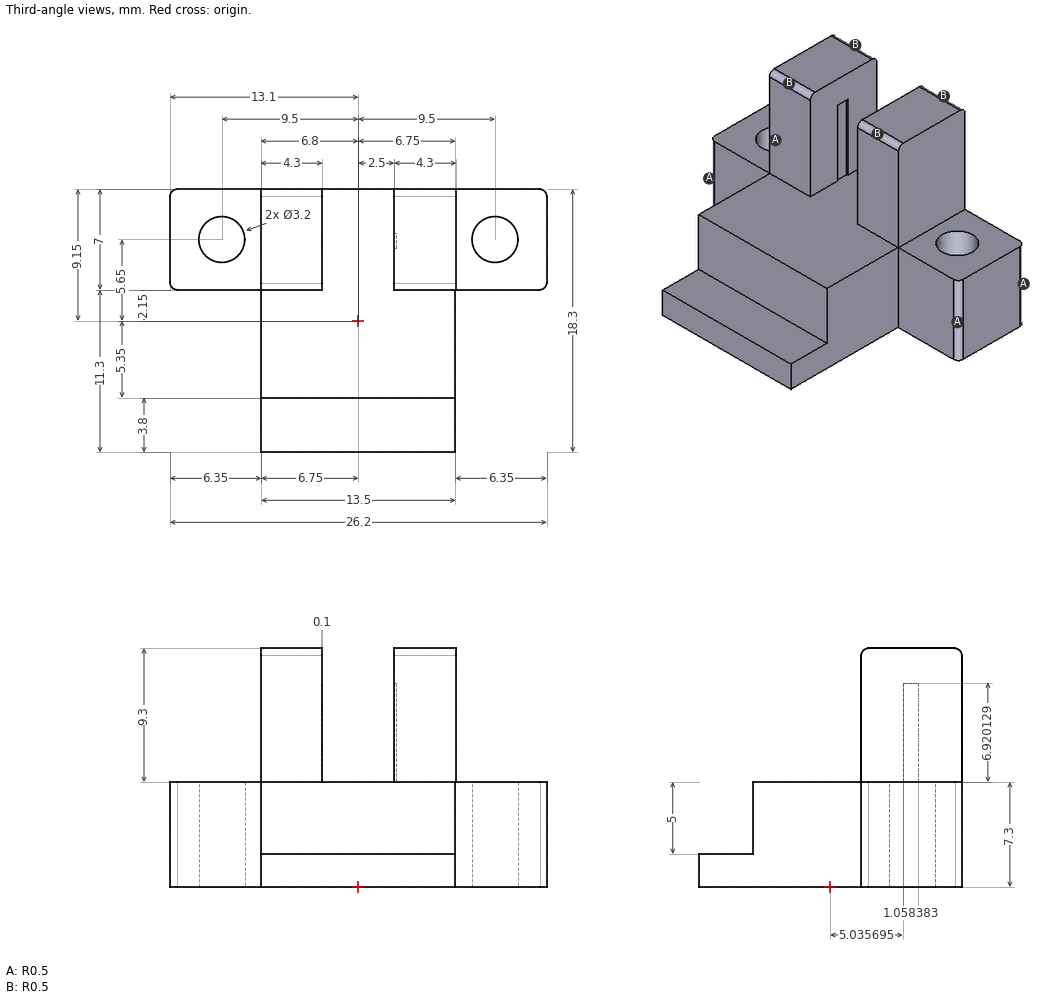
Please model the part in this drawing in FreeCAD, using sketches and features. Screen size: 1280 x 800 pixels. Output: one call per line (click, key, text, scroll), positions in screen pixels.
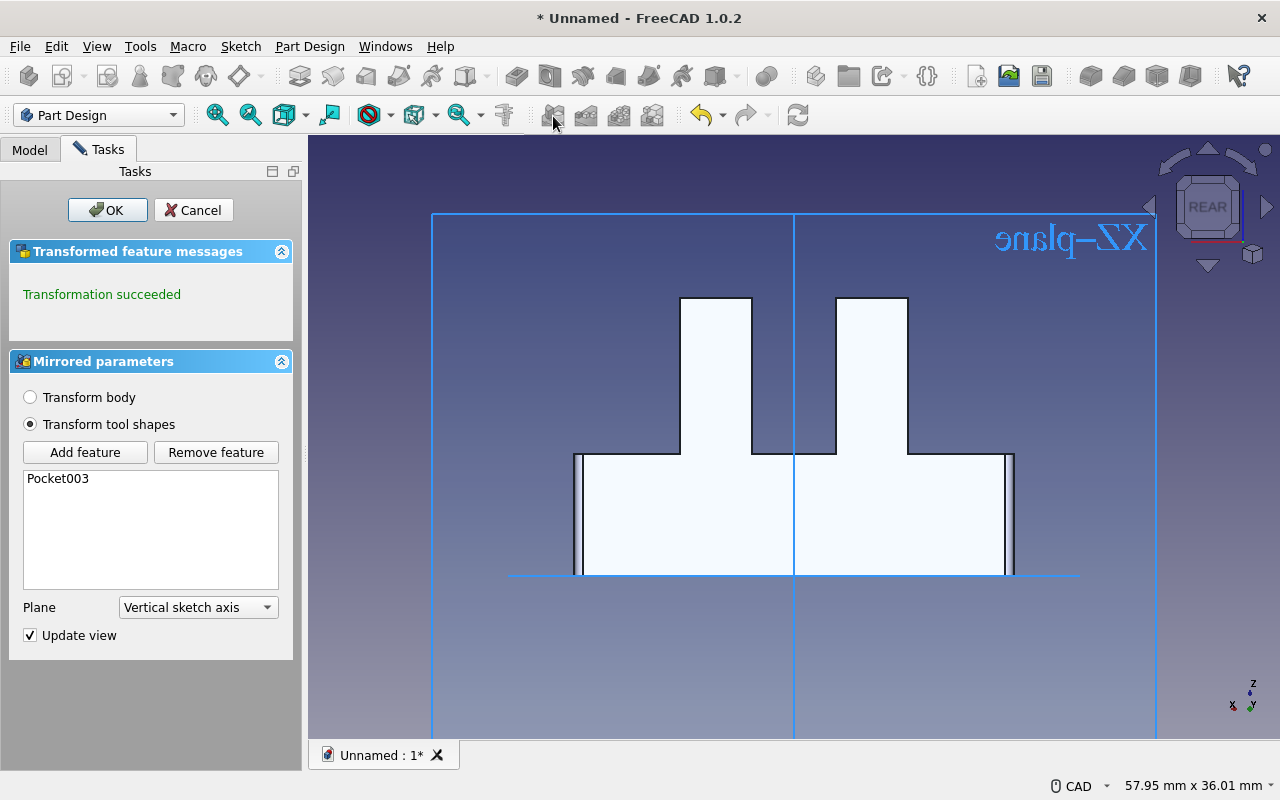
click(199, 608)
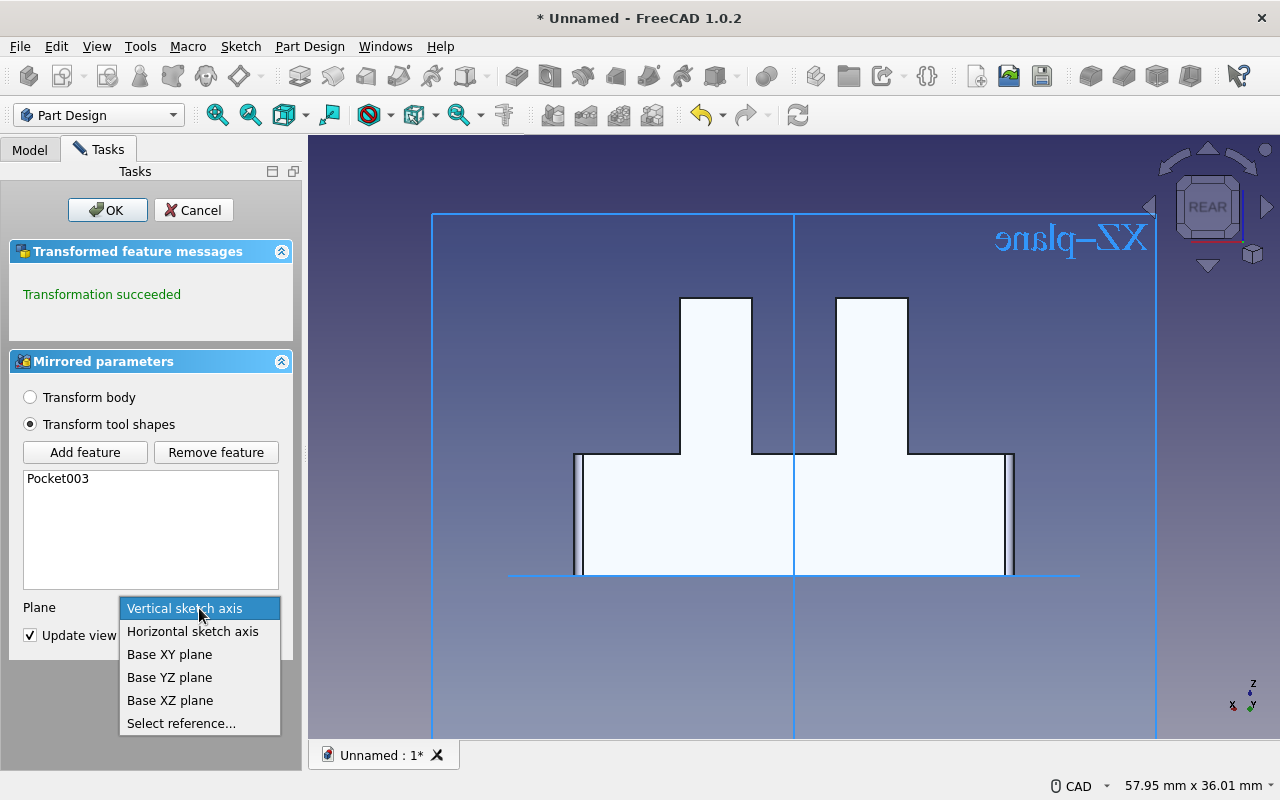
click(198, 678)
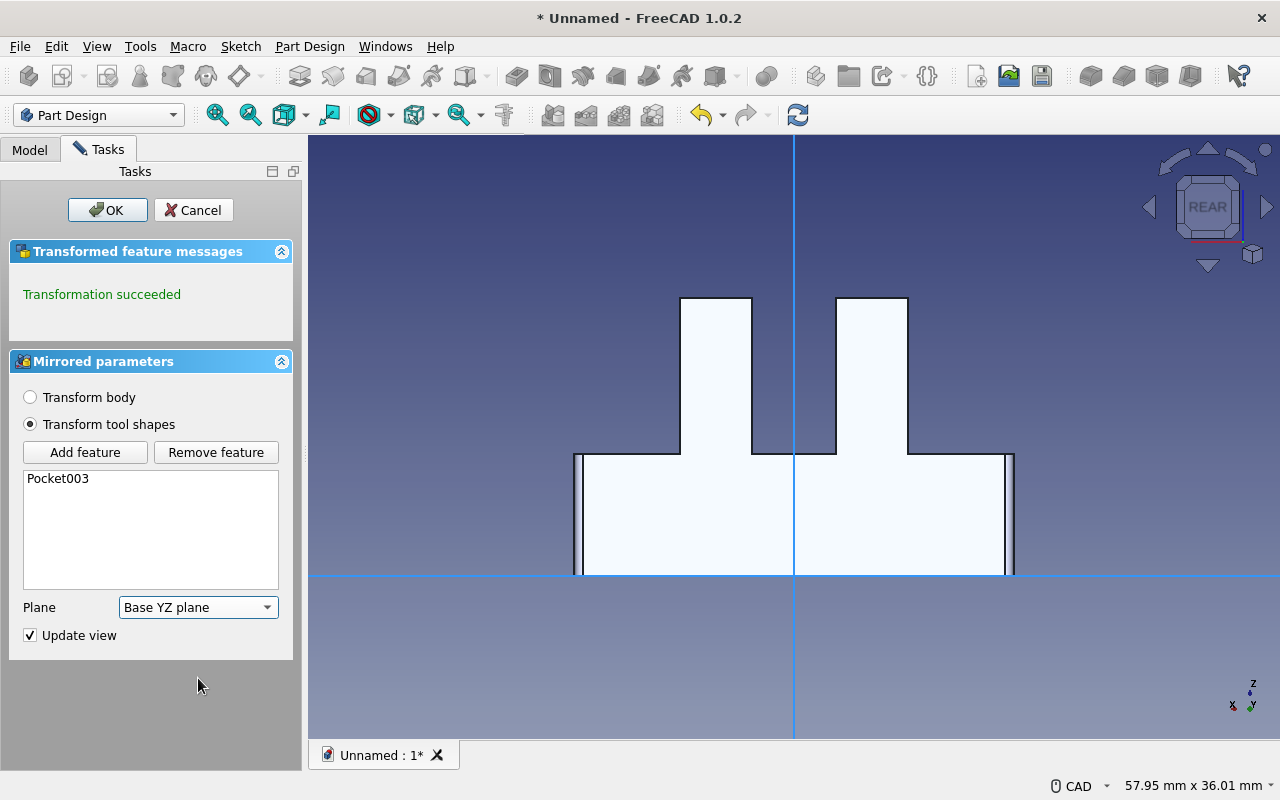
click(108, 210)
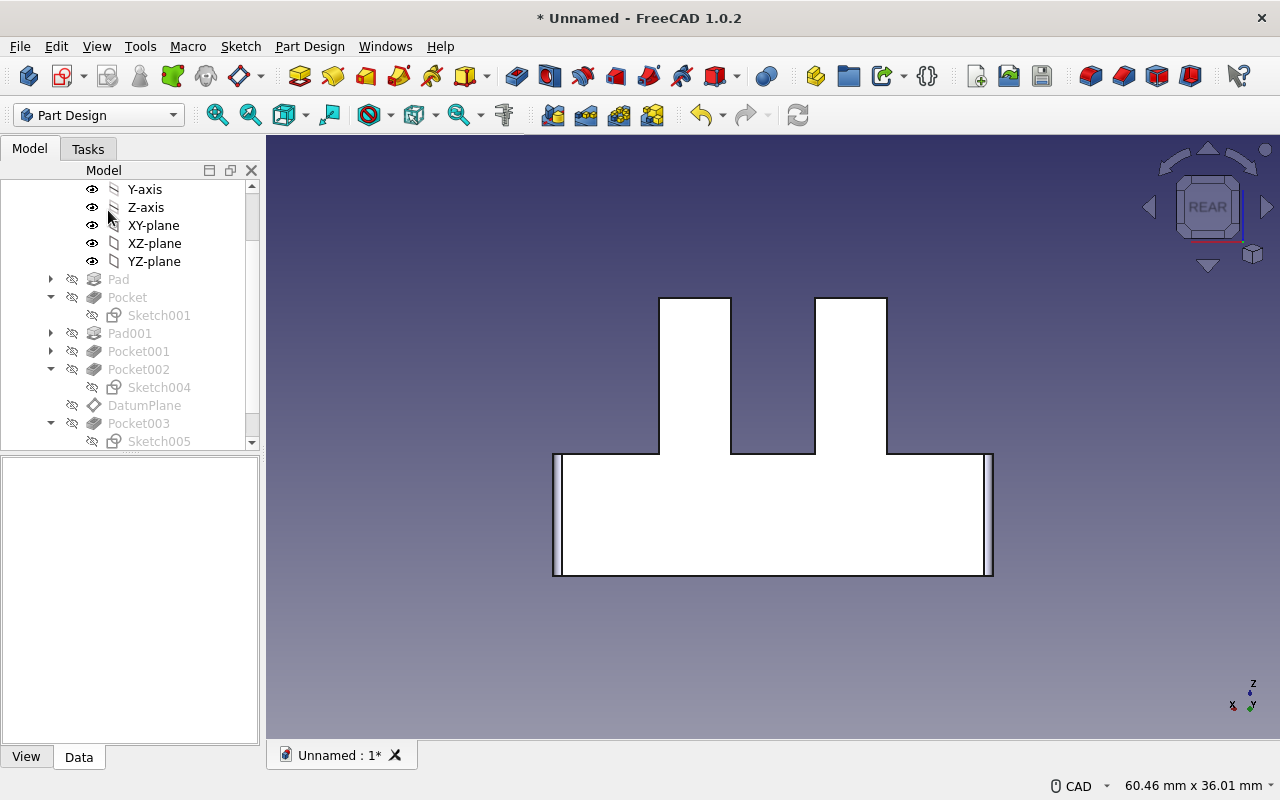
click(695, 297)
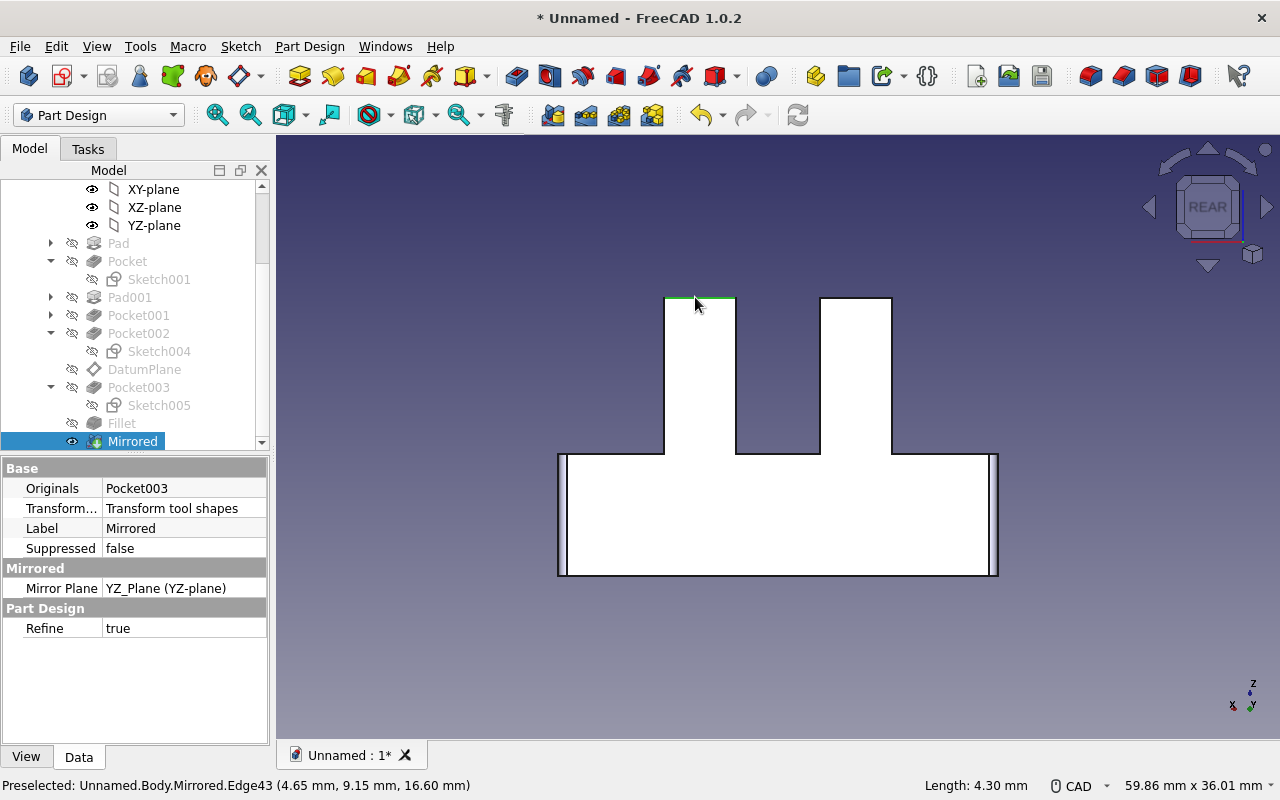
click(856, 297, ctrl)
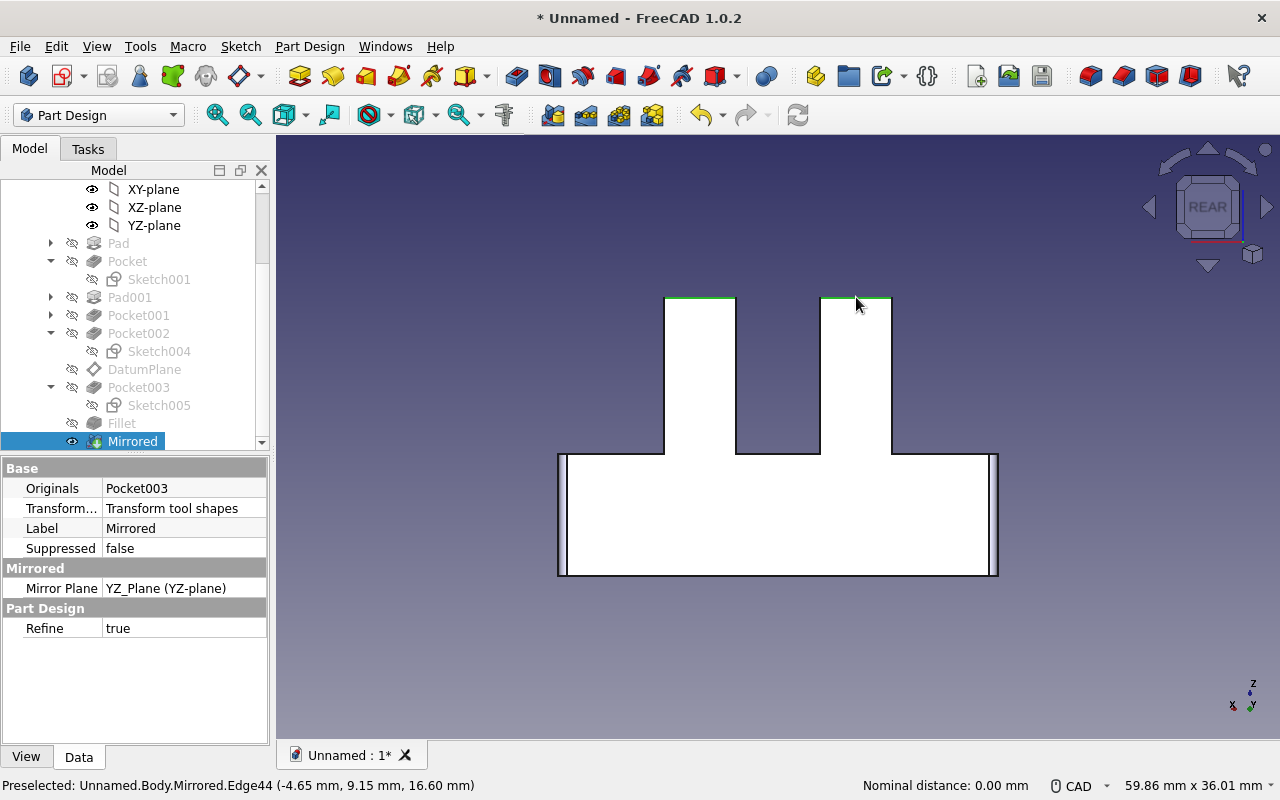
key(0)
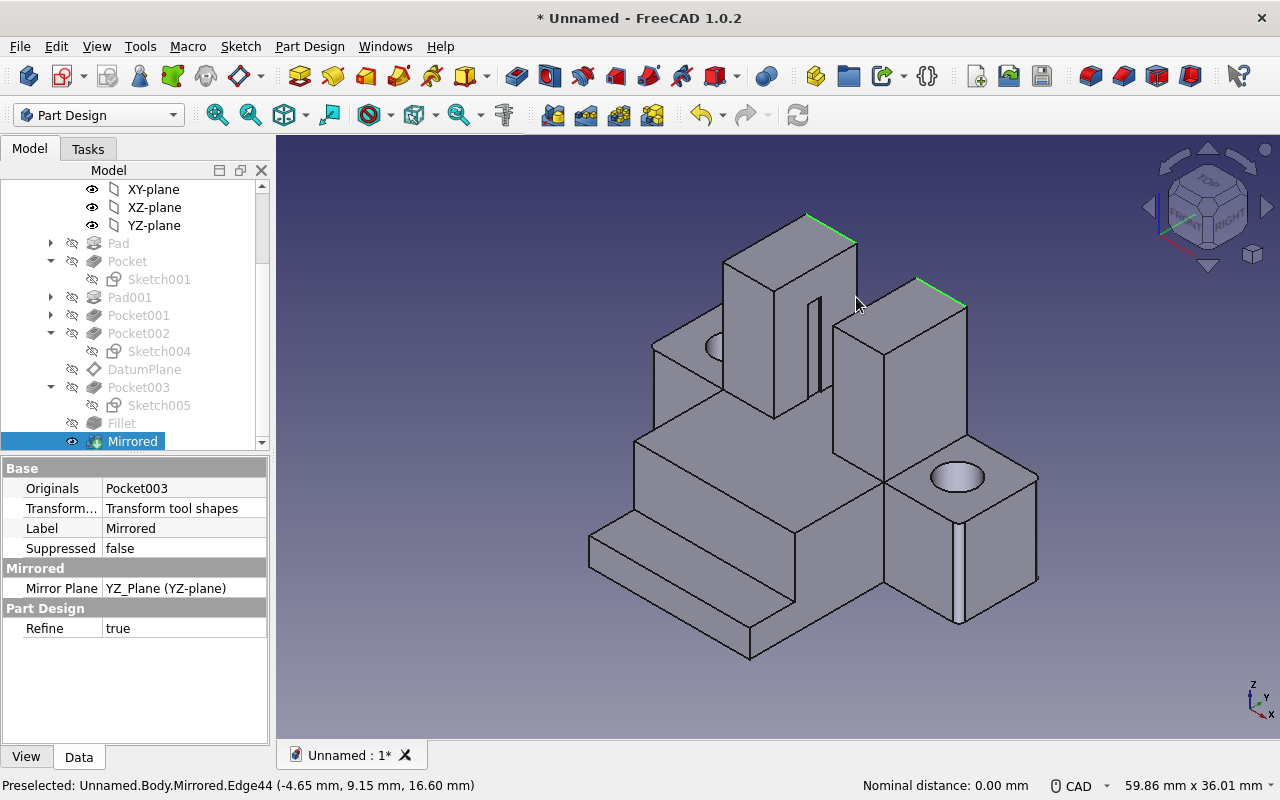
click(859, 339, ctrl)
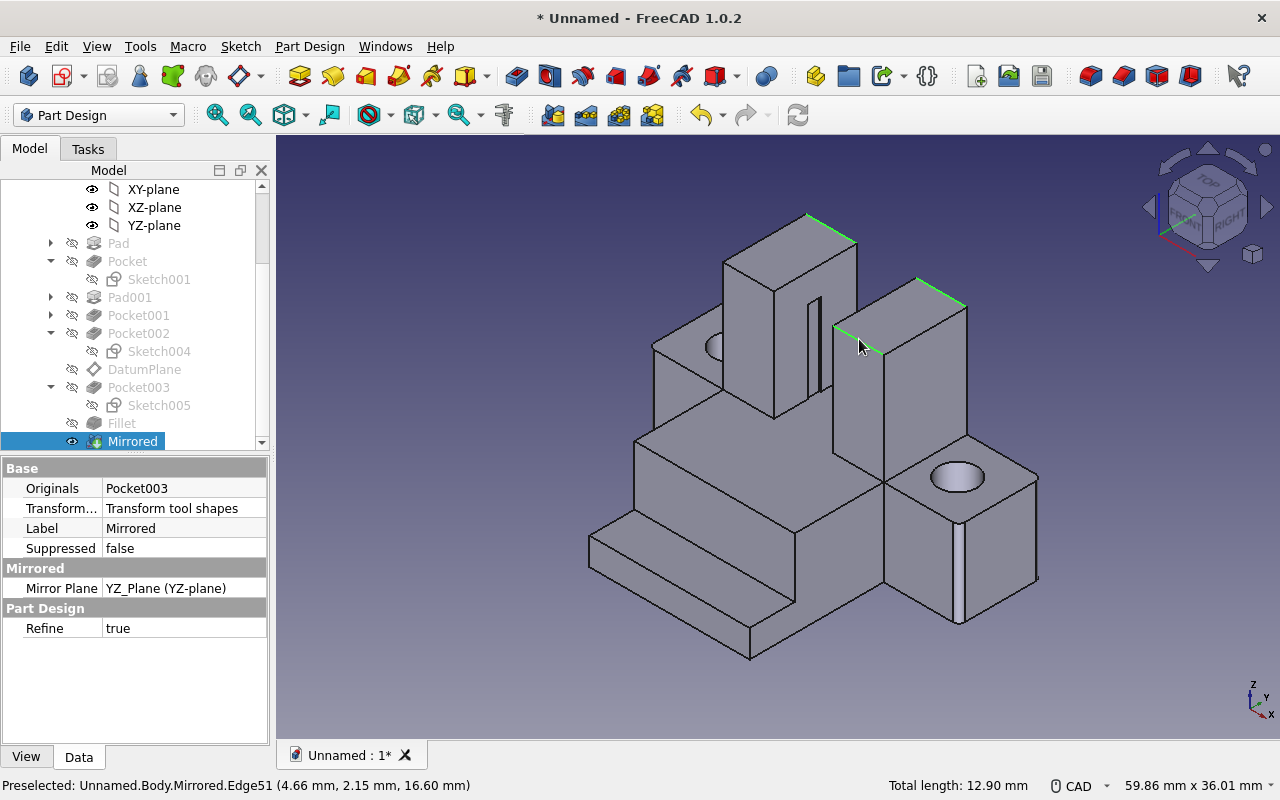
click(748, 276, ctrl)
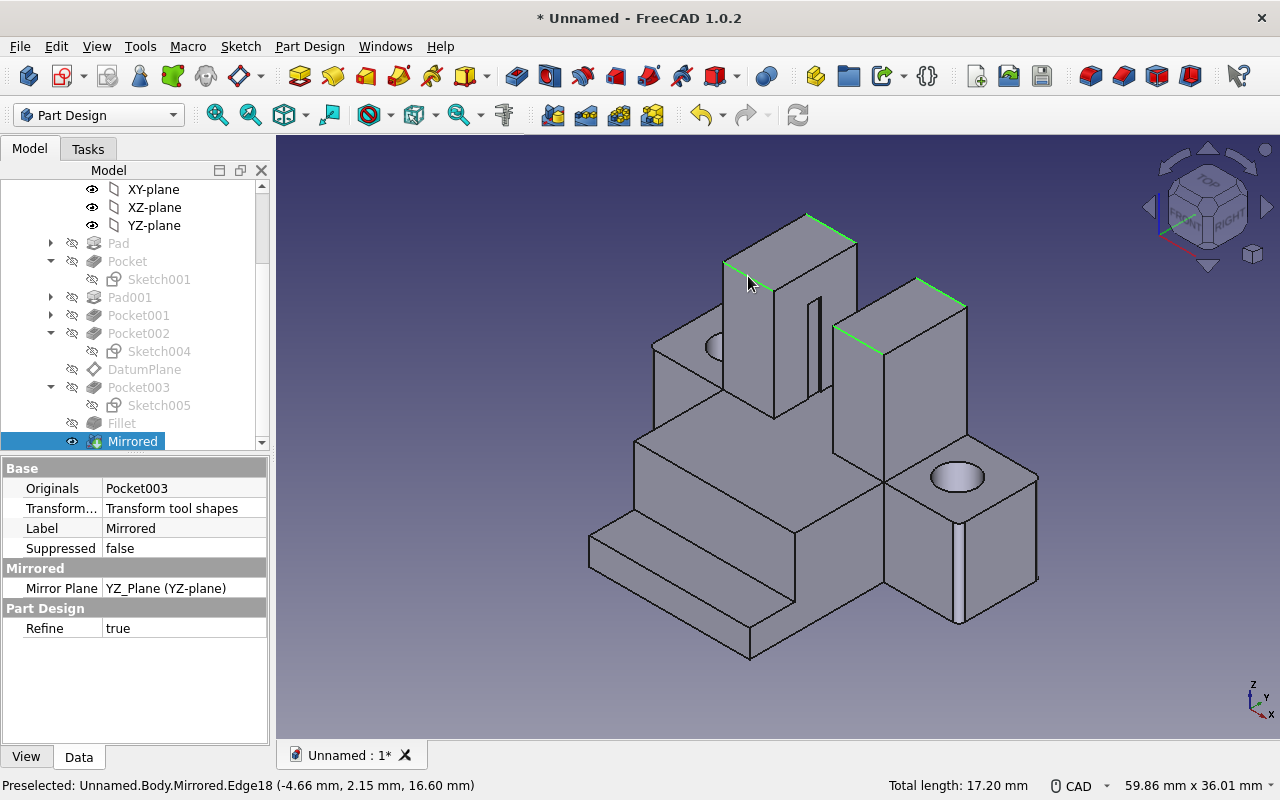
click(1091, 76)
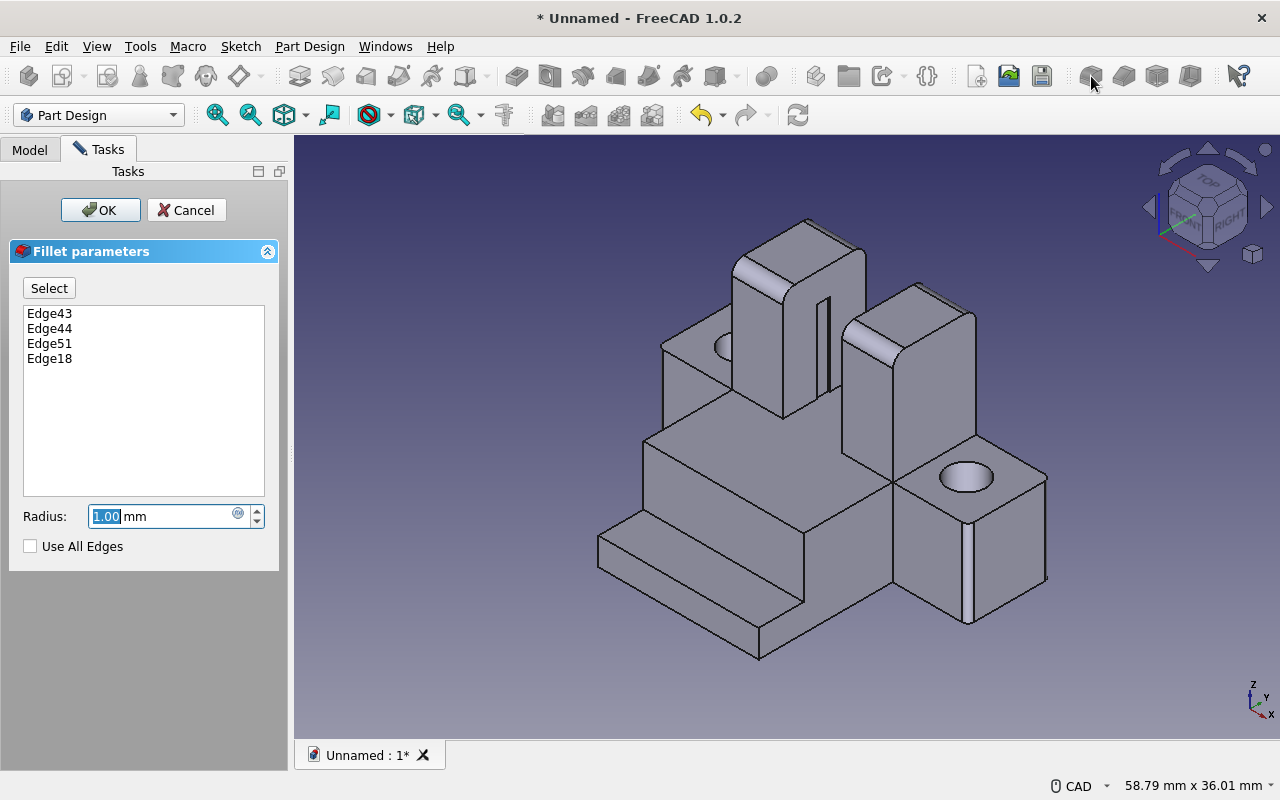
text(0.5)
key(Tab)